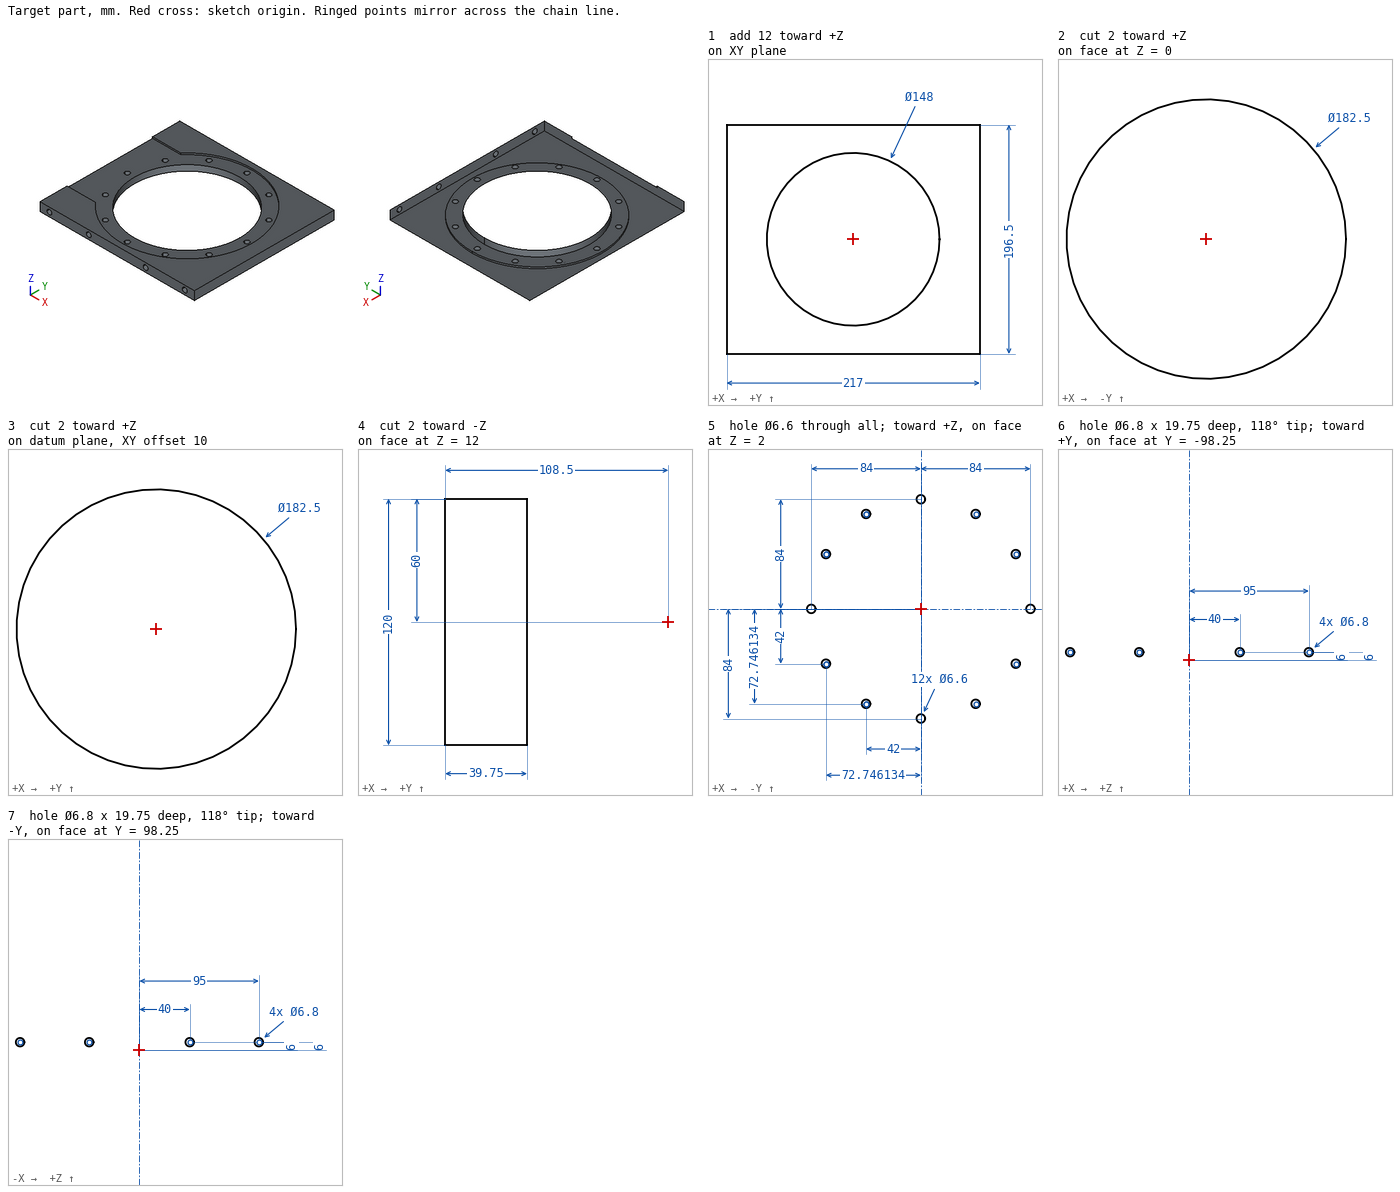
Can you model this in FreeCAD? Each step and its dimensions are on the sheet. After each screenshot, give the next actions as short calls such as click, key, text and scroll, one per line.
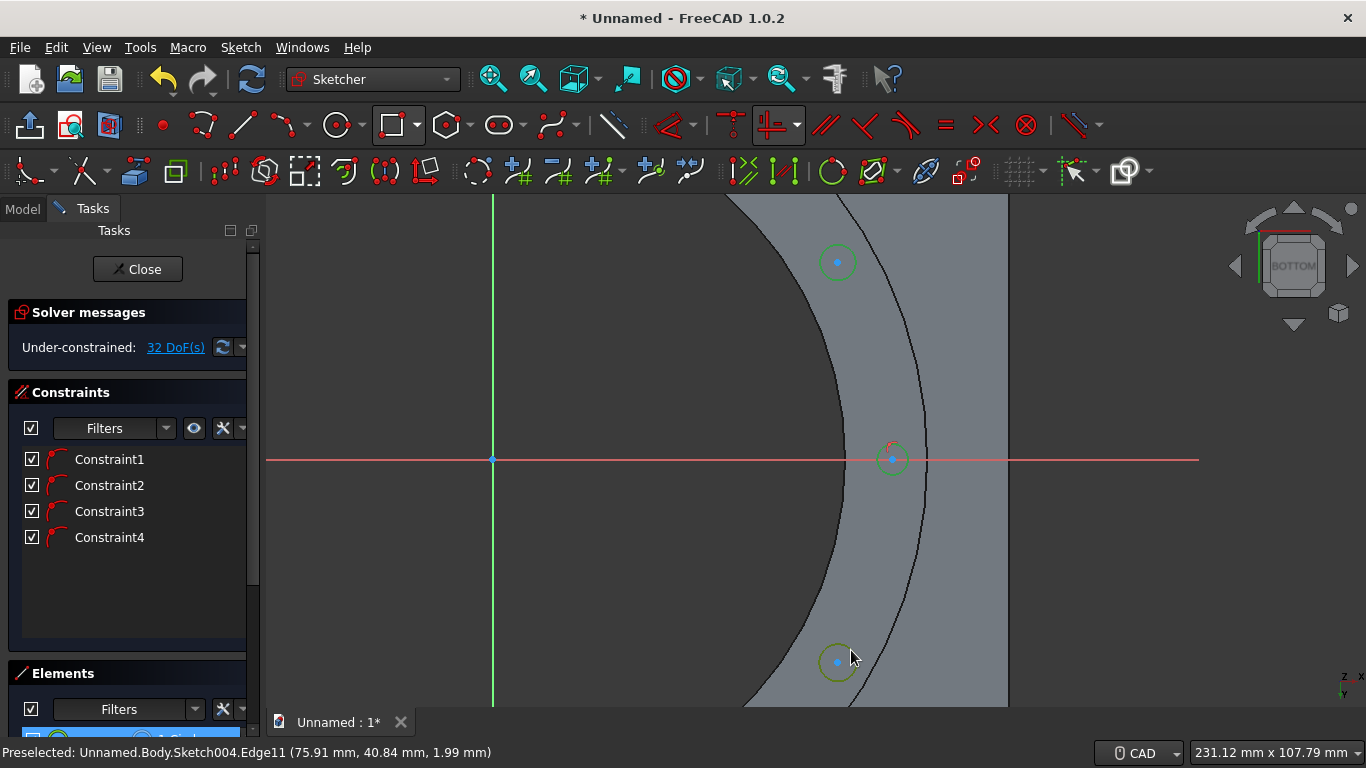
scroll(896, 445, down, 5)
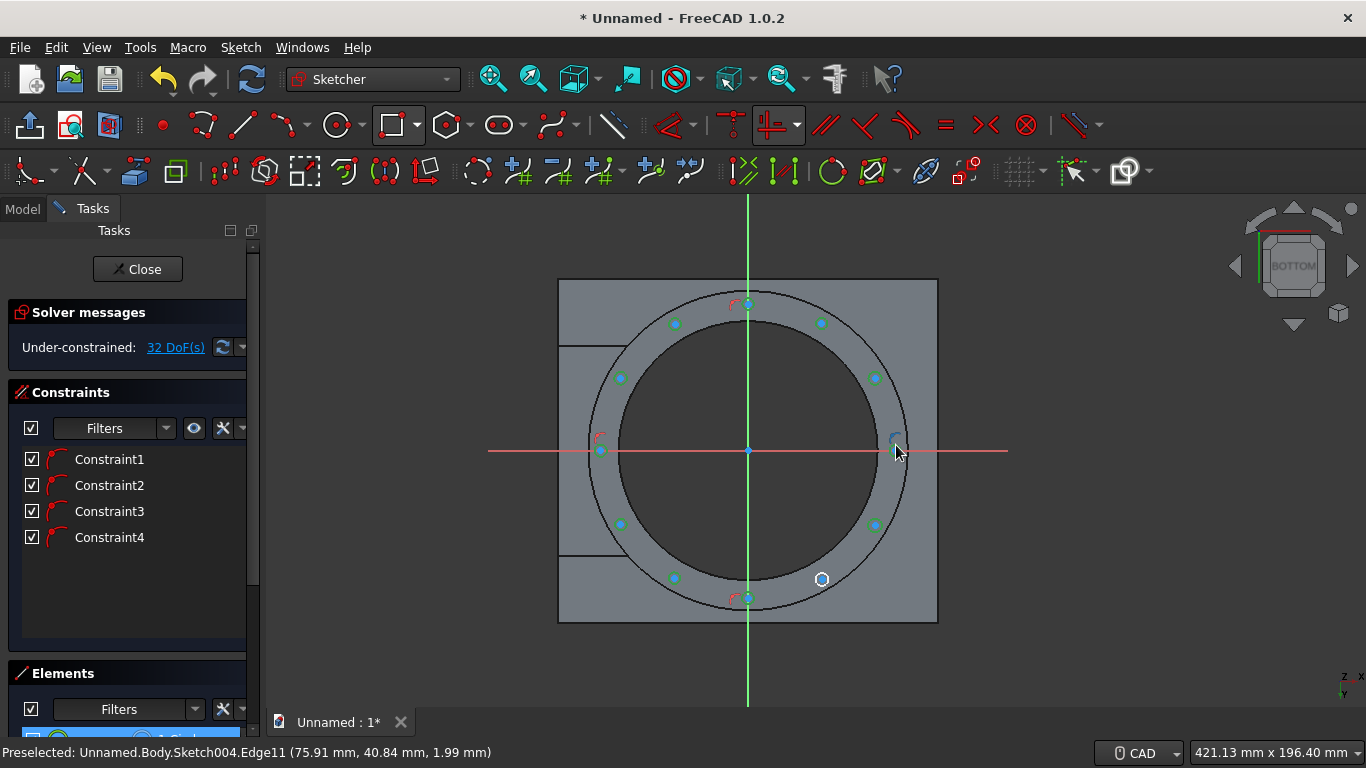
scroll(827, 575, up, 4)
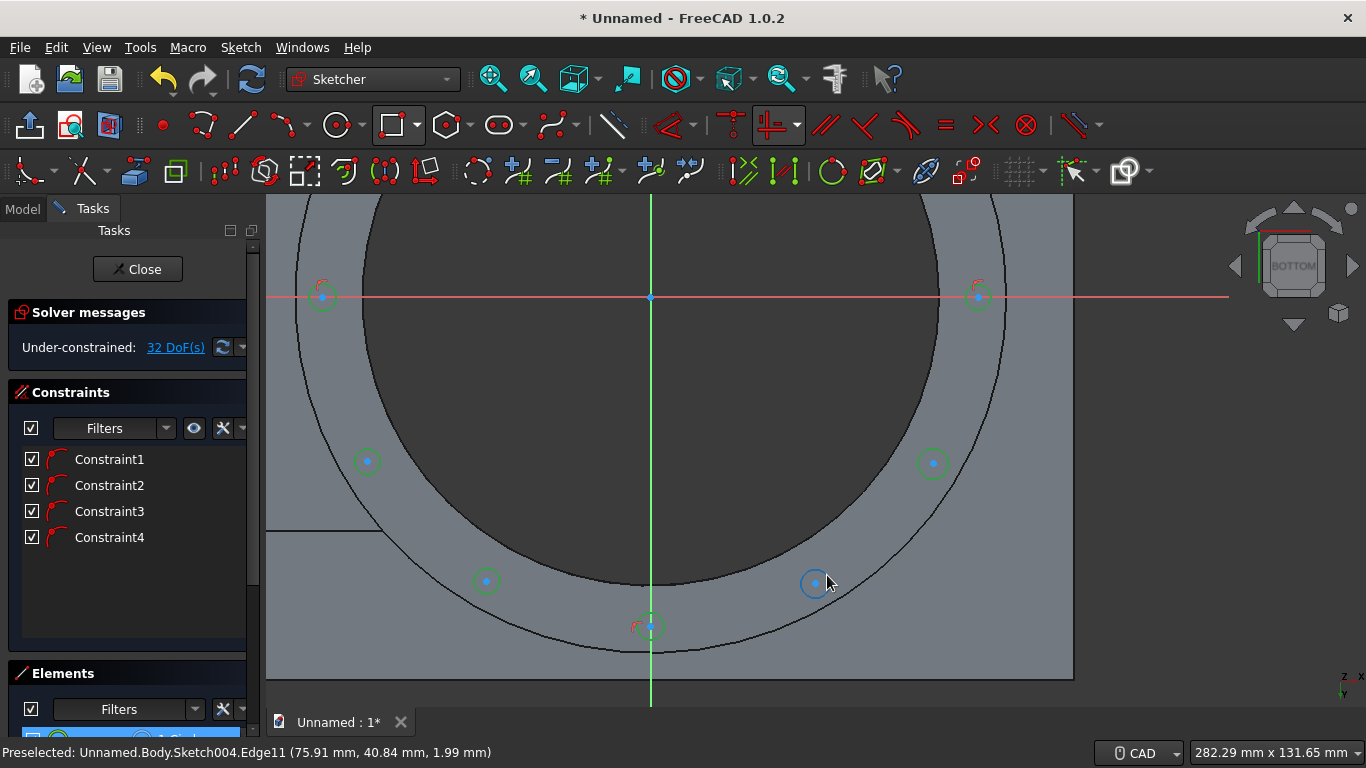
click(825, 574)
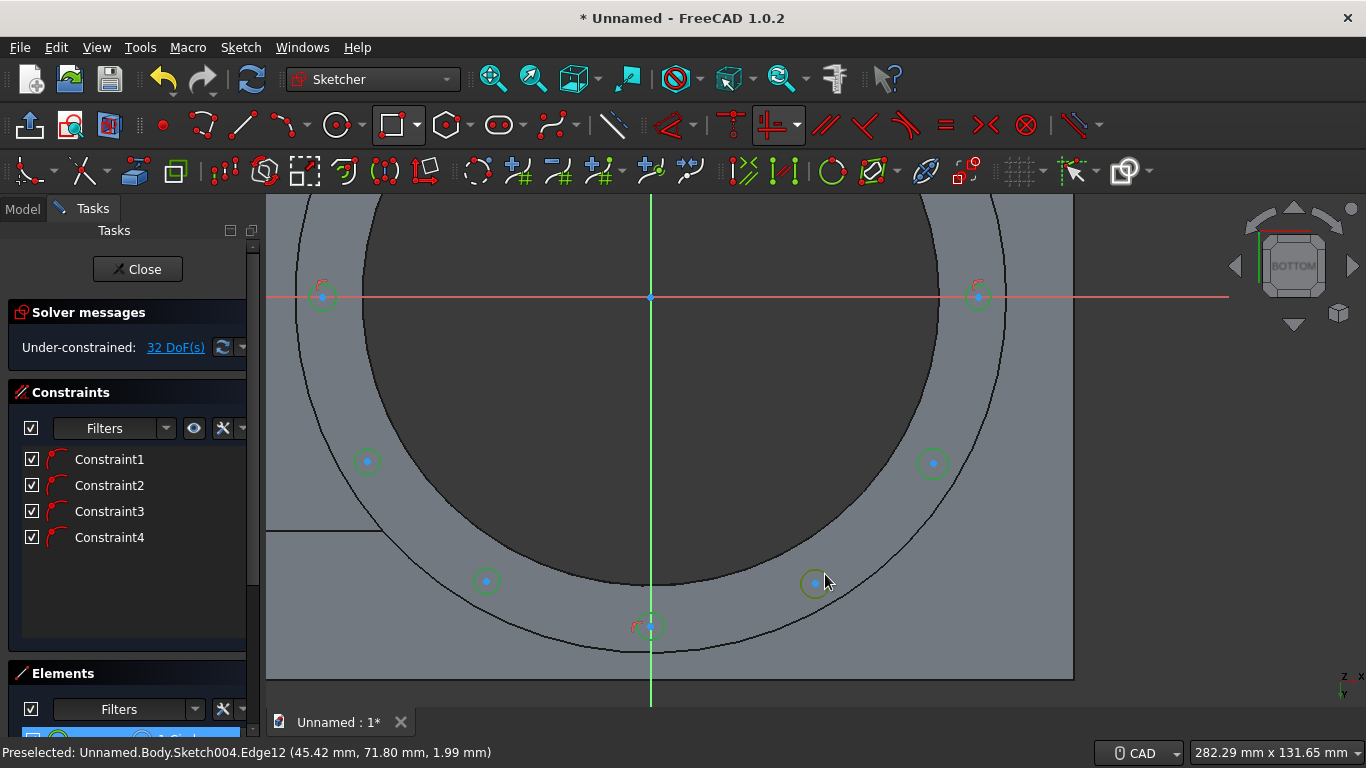
click(946, 126)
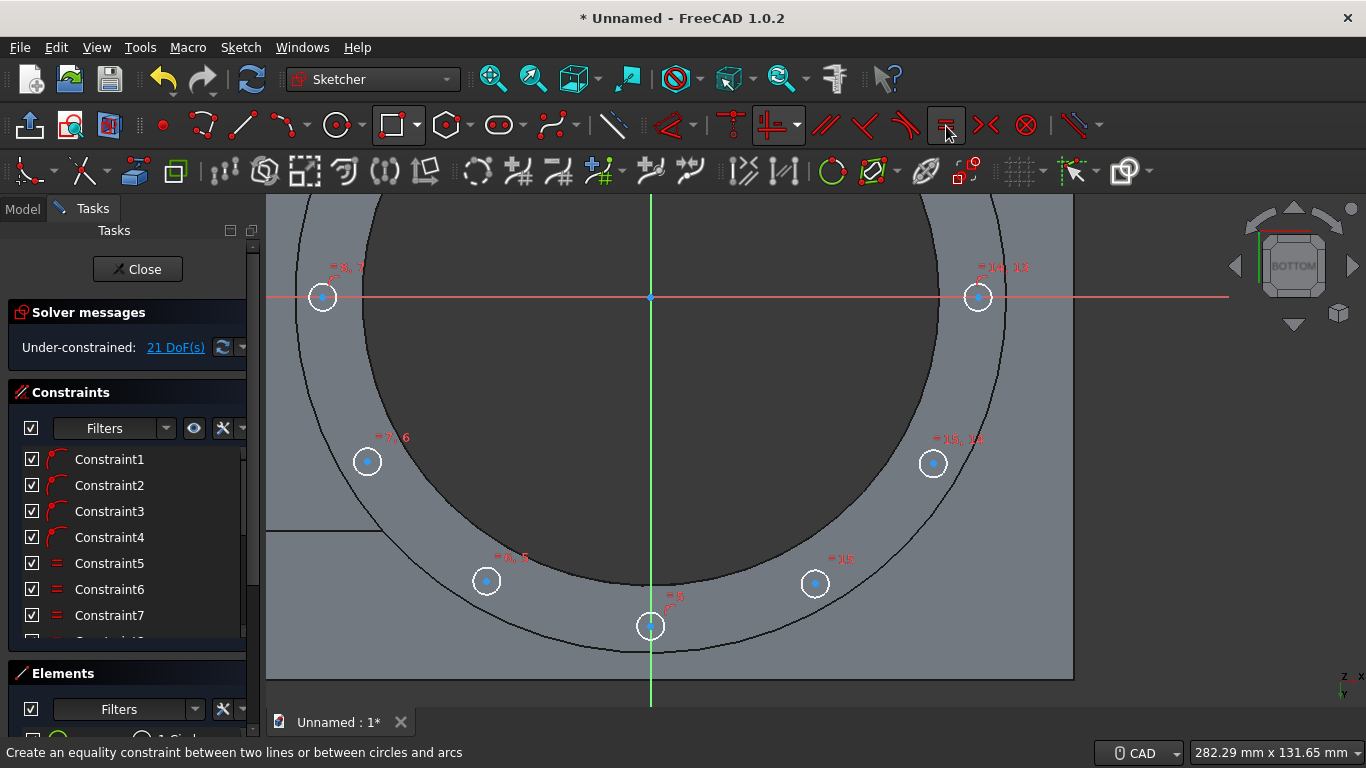
click(368, 462)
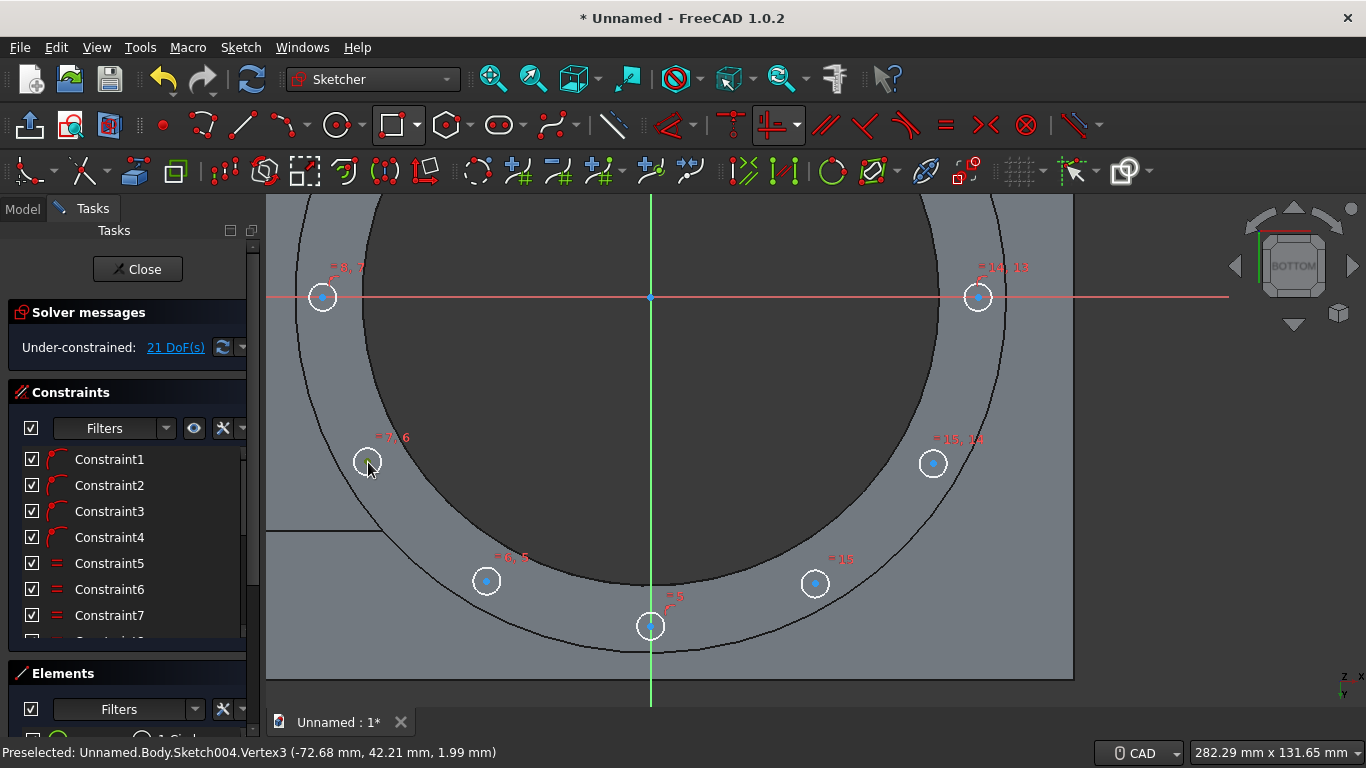
scroll(826, 575, down, 4)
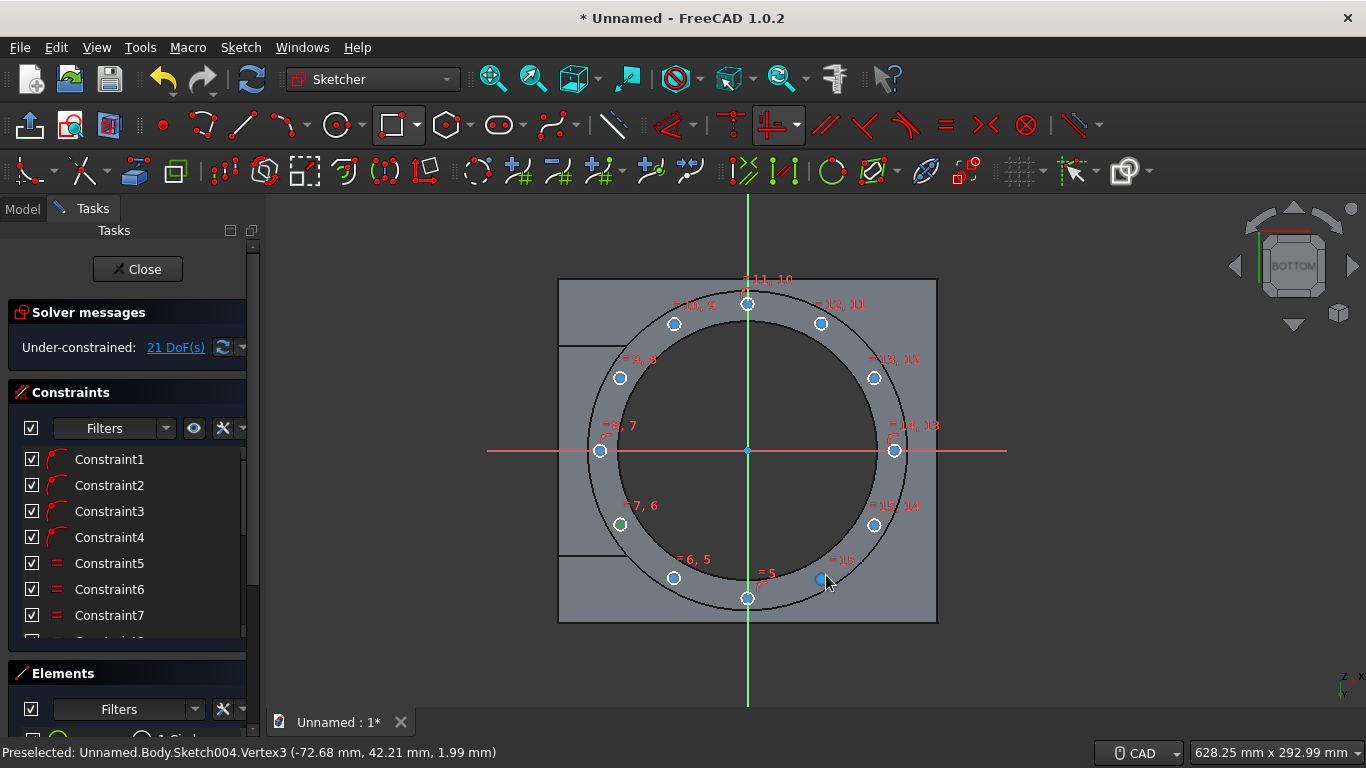
click(620, 378)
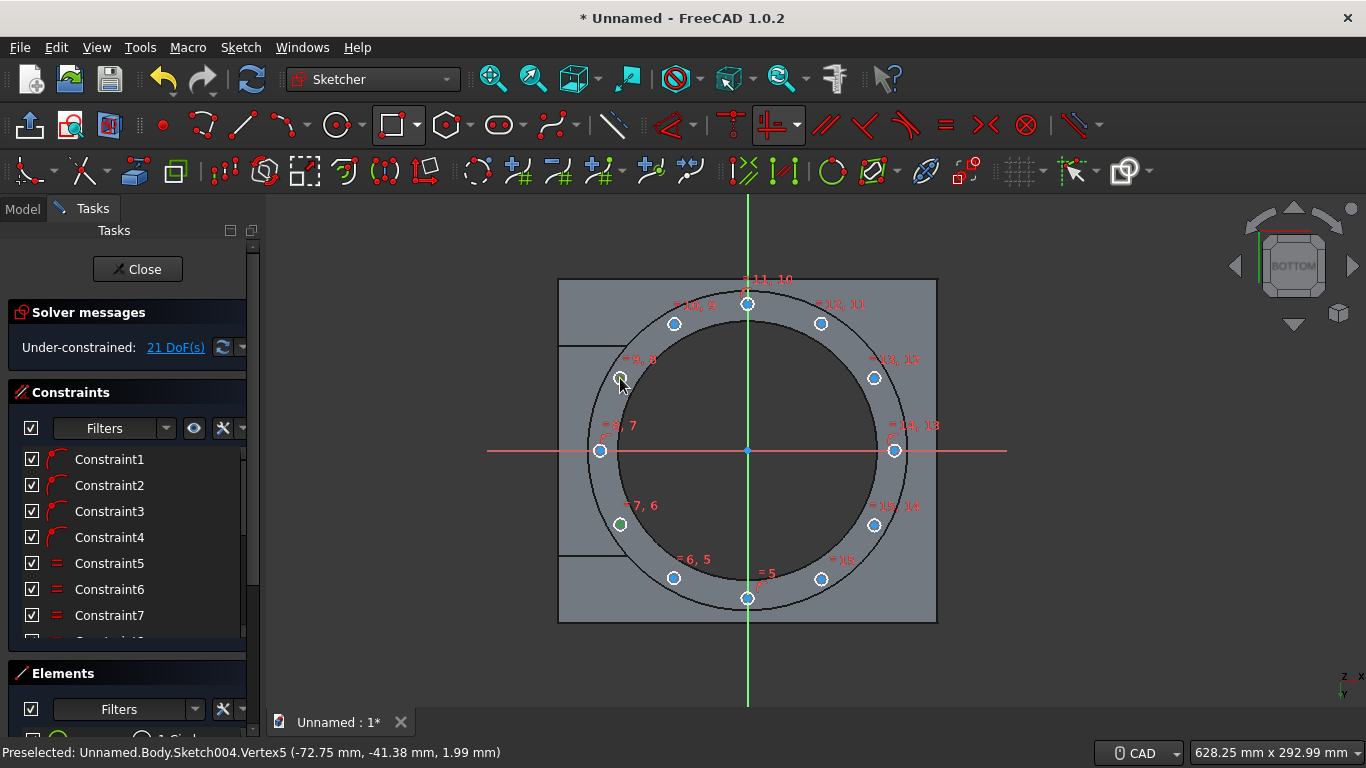
click(488, 451)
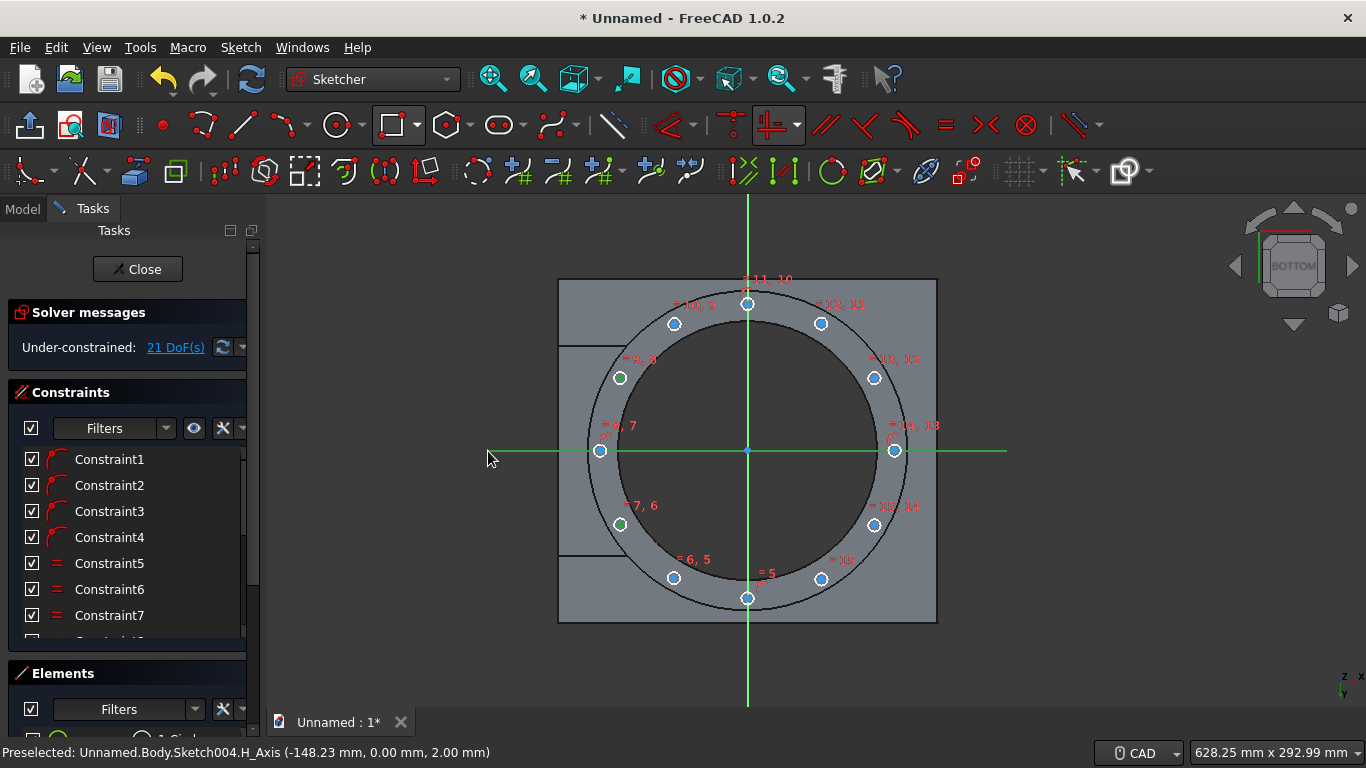
click(986, 126)